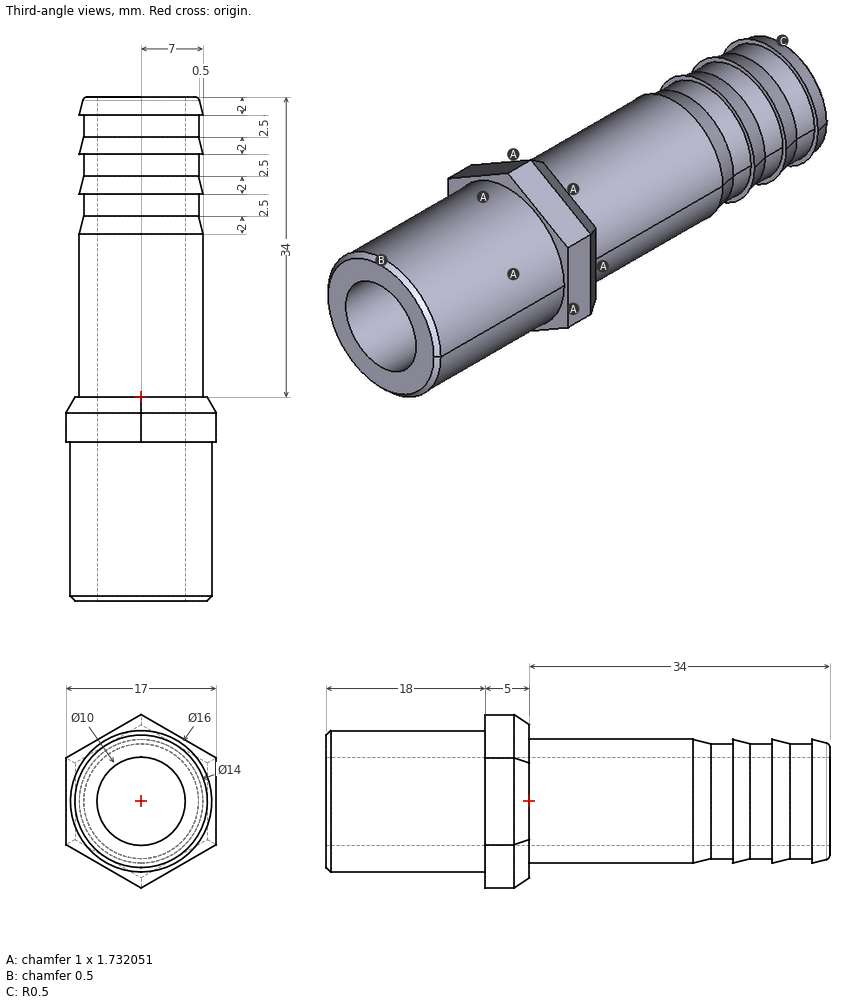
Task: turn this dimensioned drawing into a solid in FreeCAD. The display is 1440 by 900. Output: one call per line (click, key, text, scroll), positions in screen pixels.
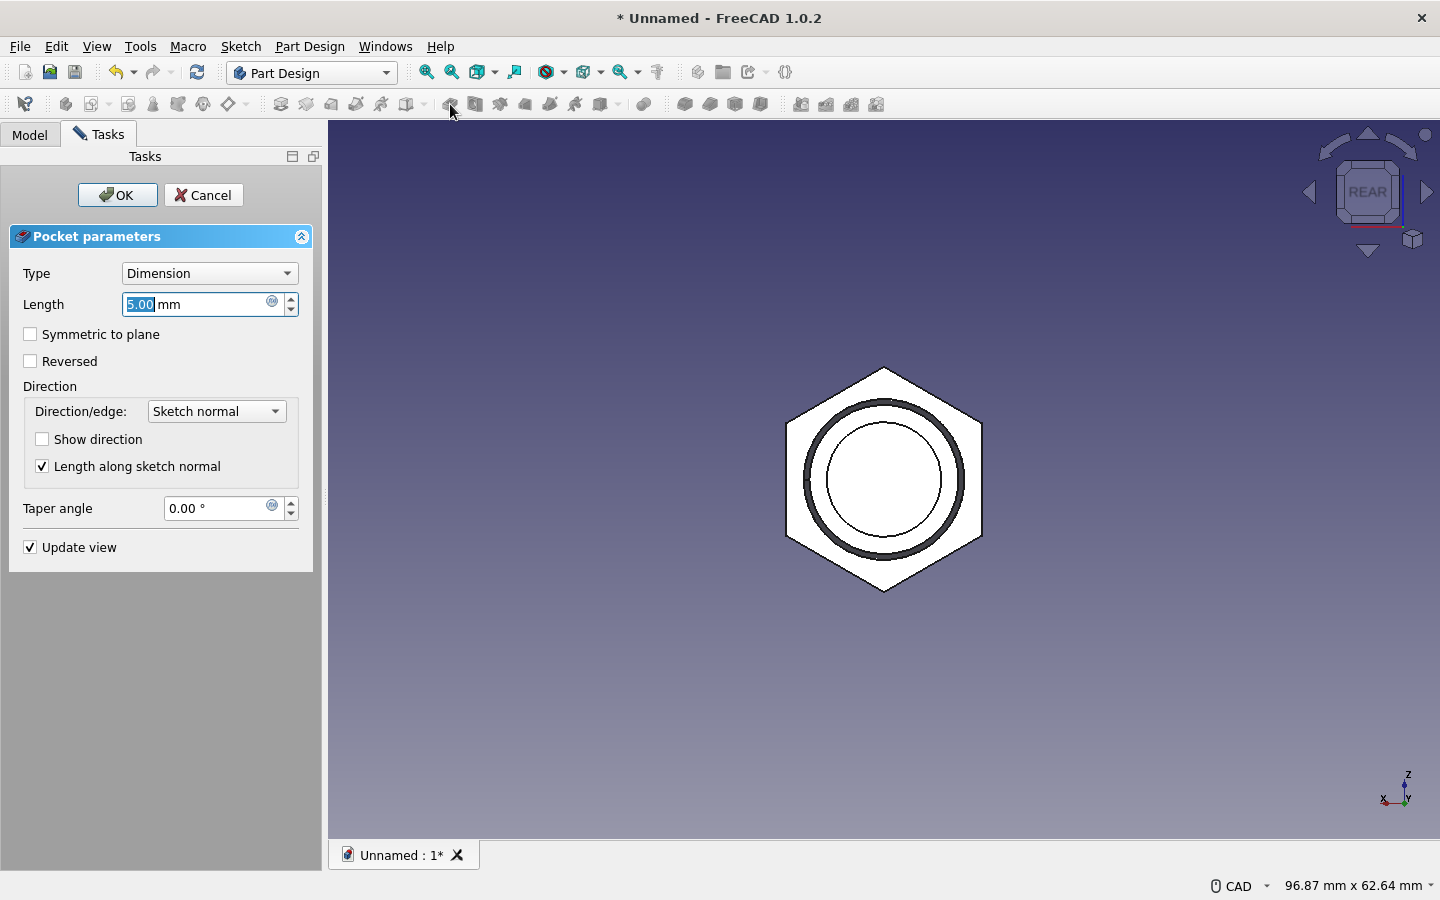
click(210, 274)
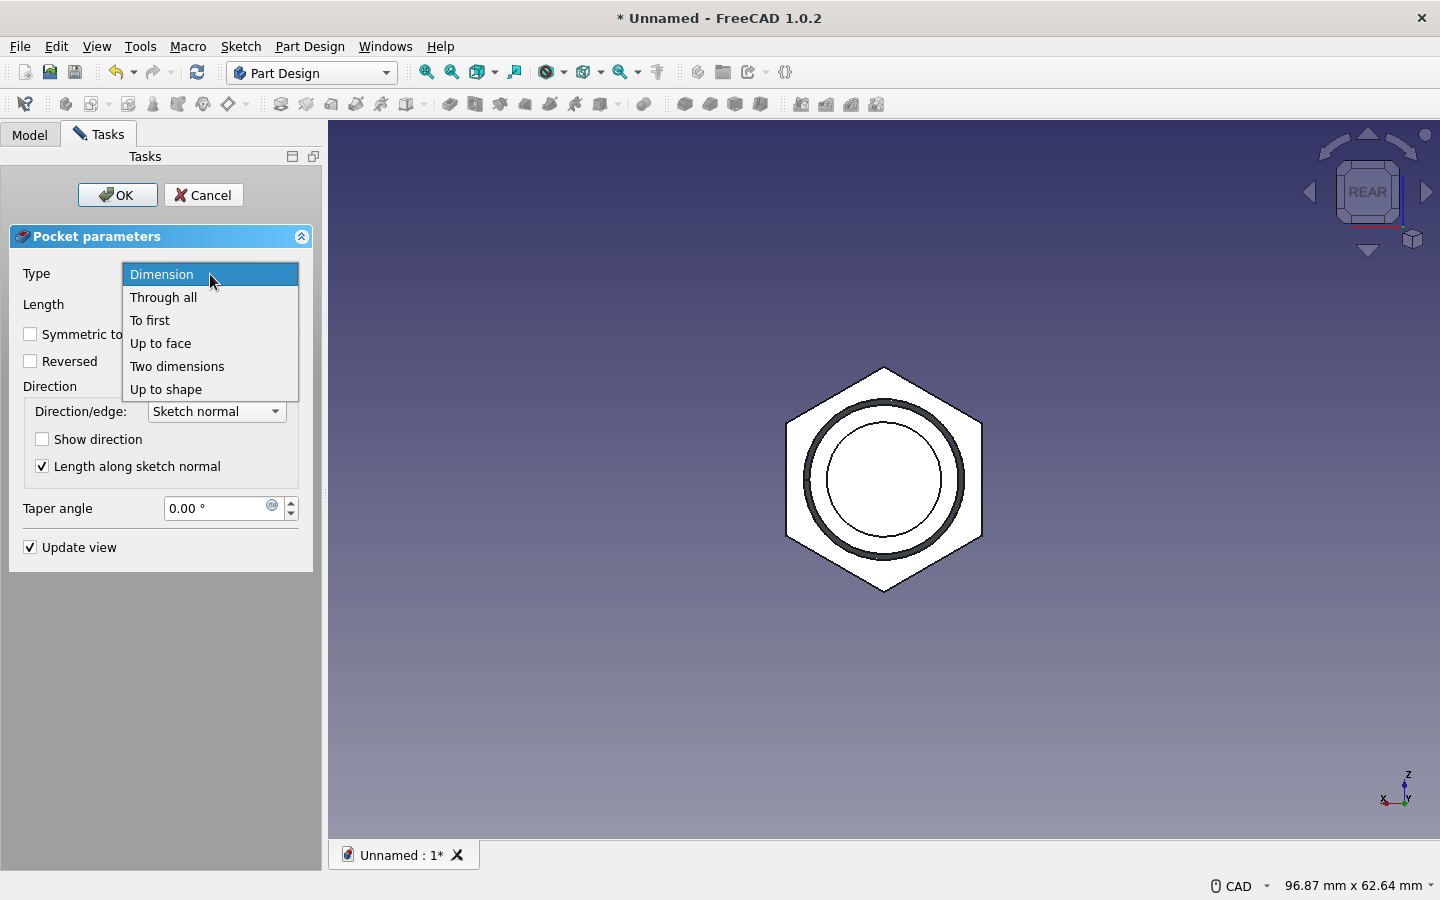
click(208, 298)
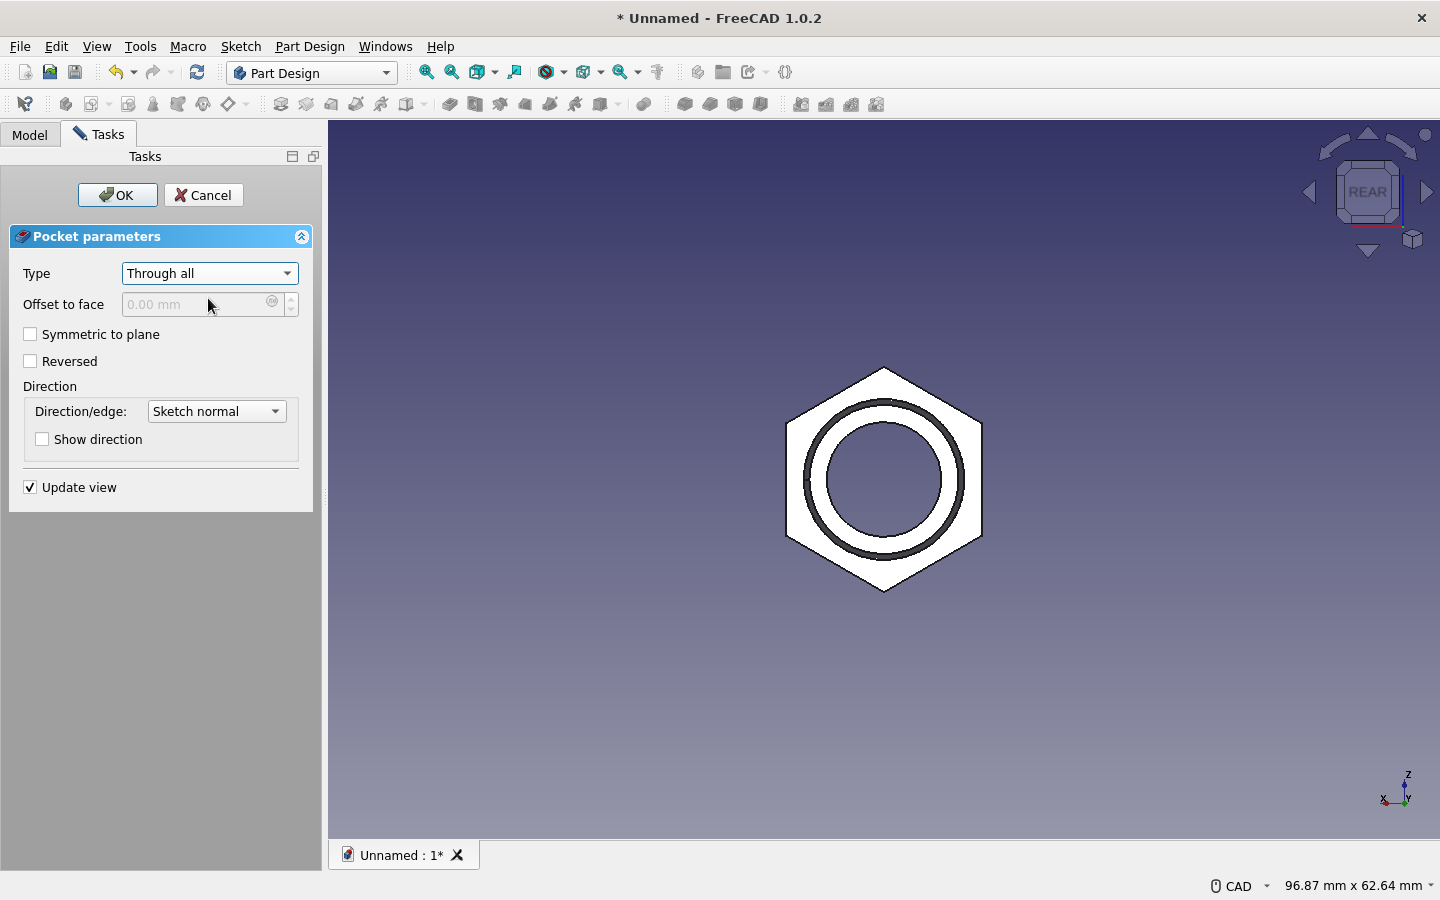
click(118, 195)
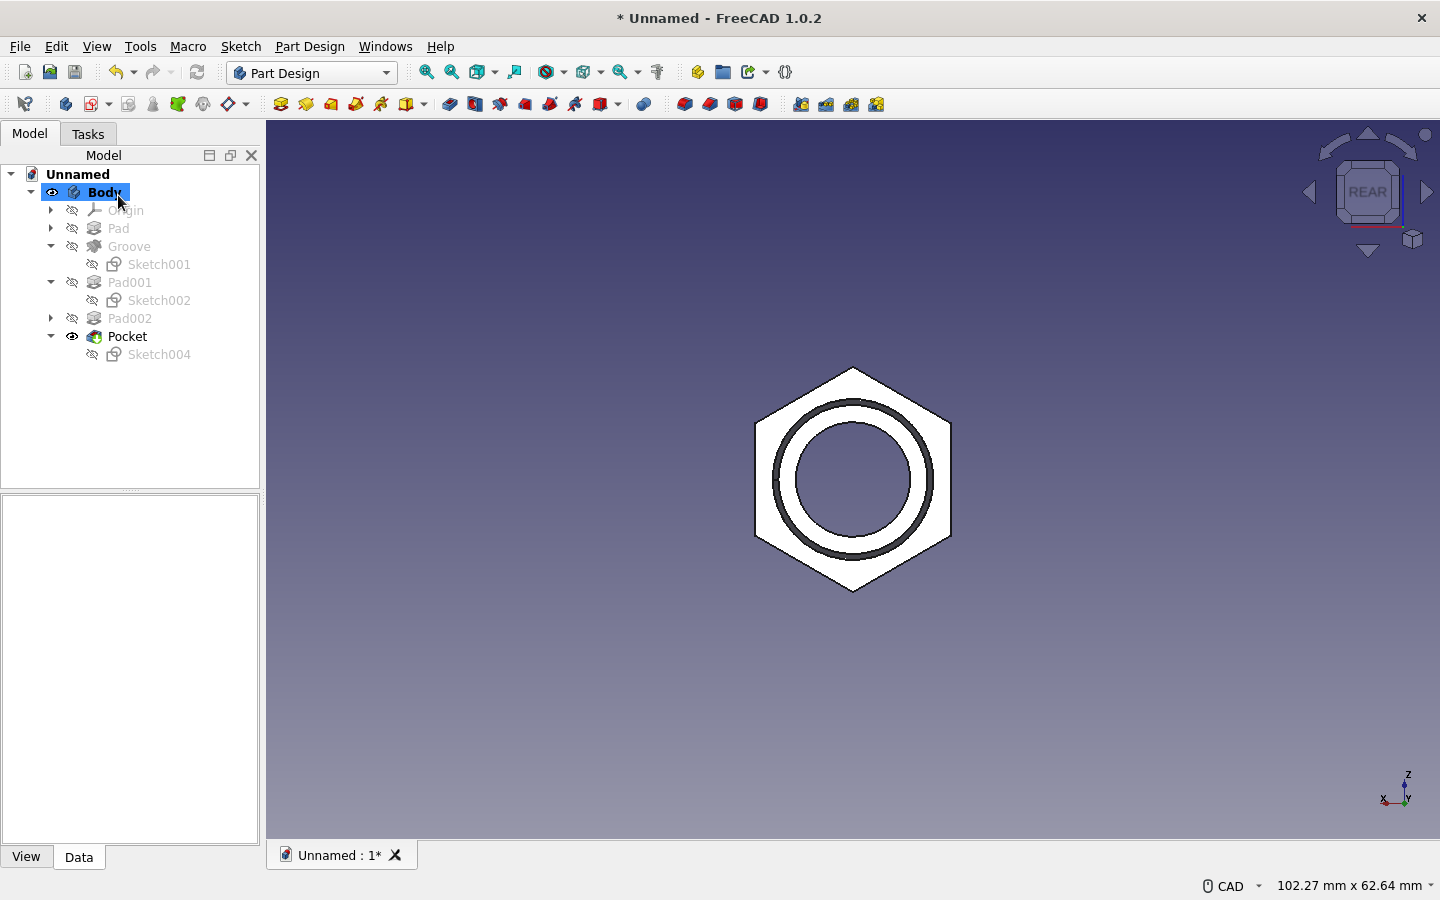
click(427, 72)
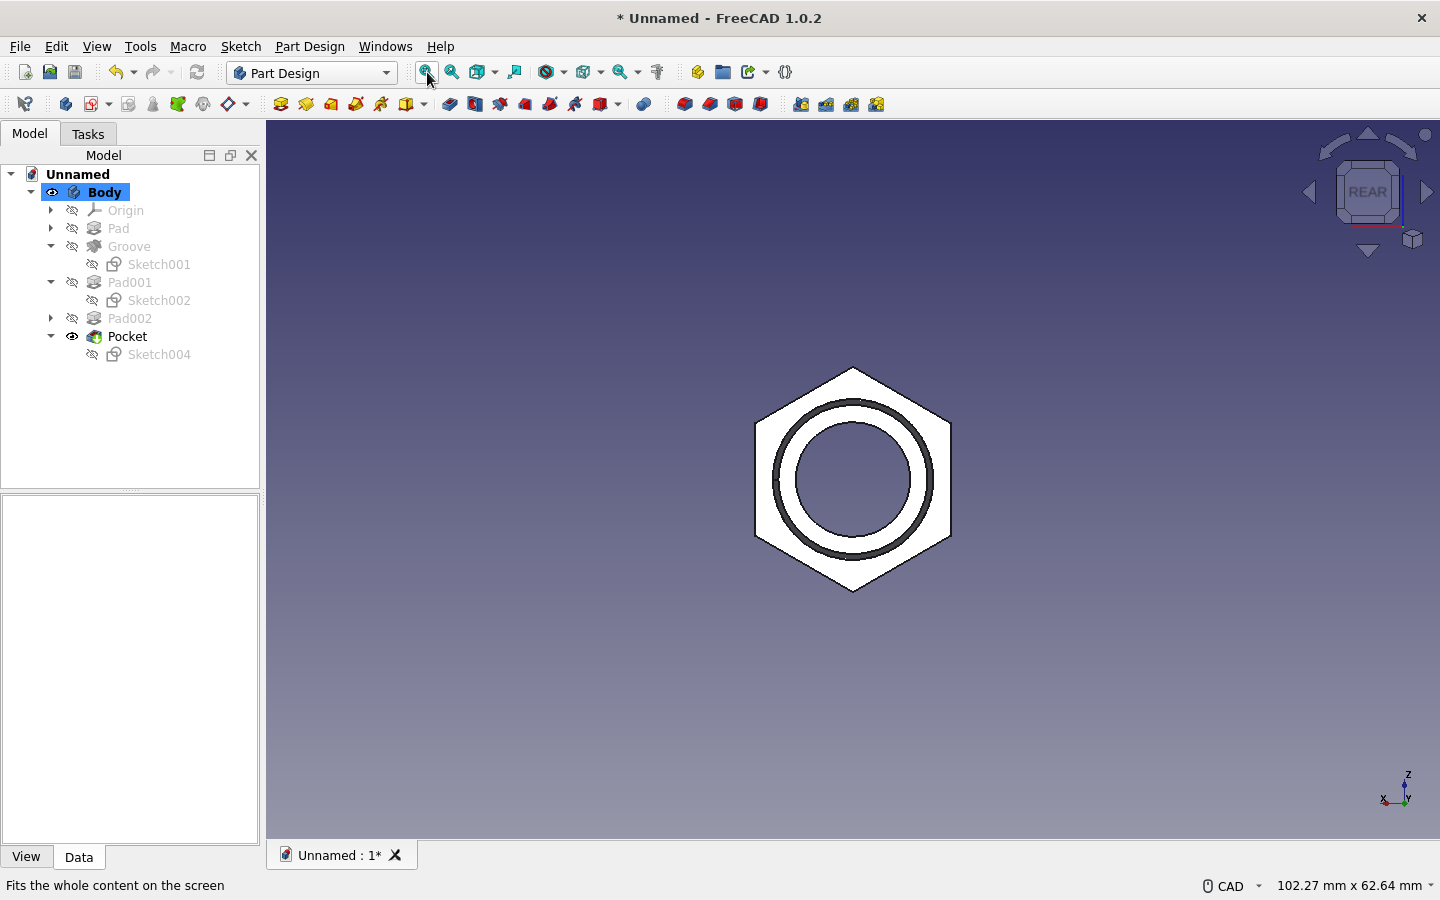
click(804, 563)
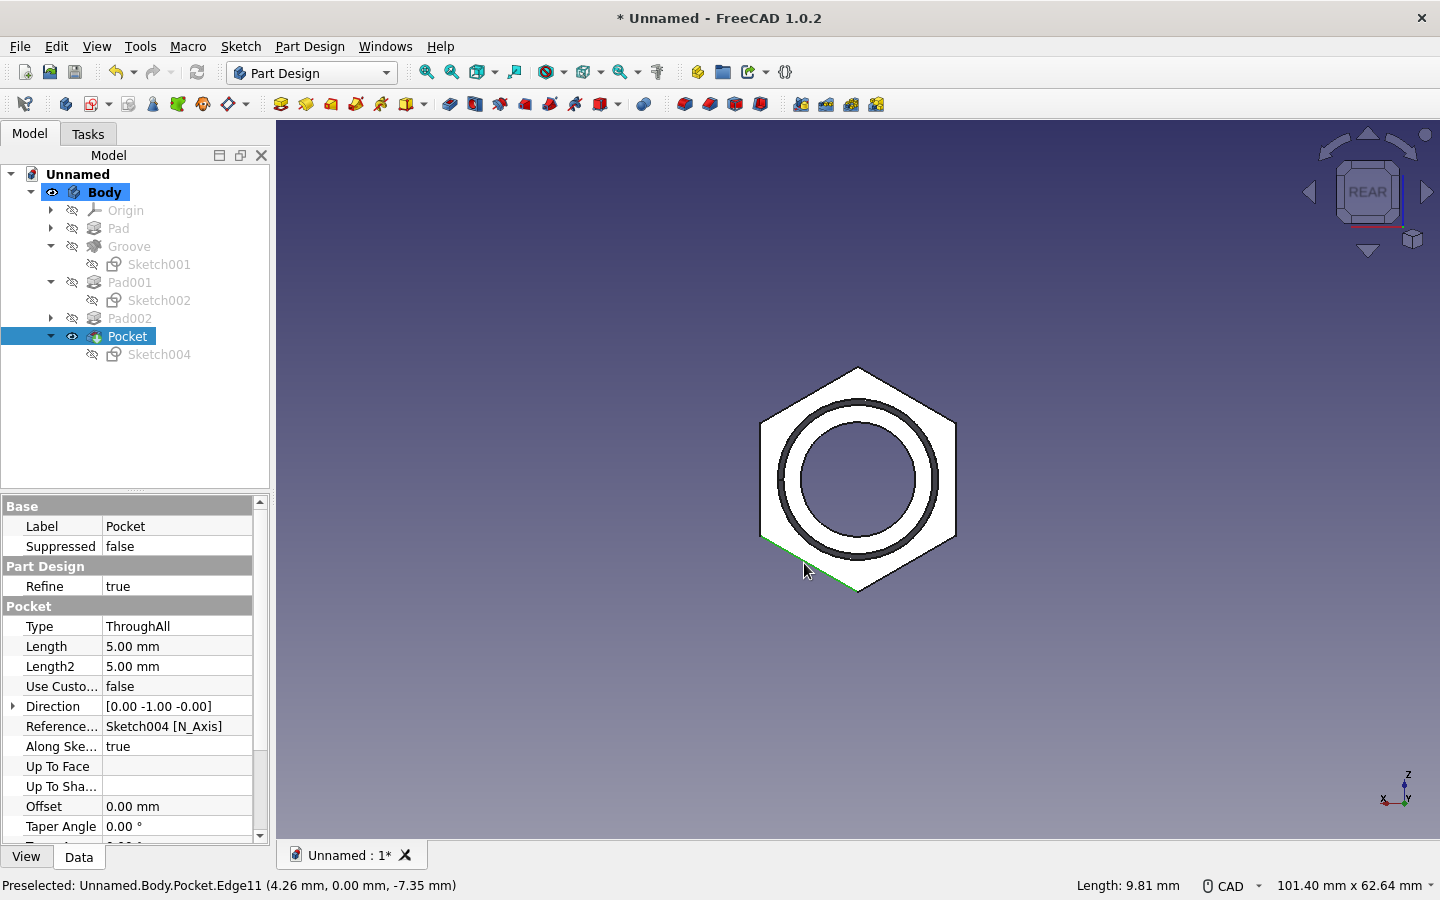
click(956, 478, ctrl)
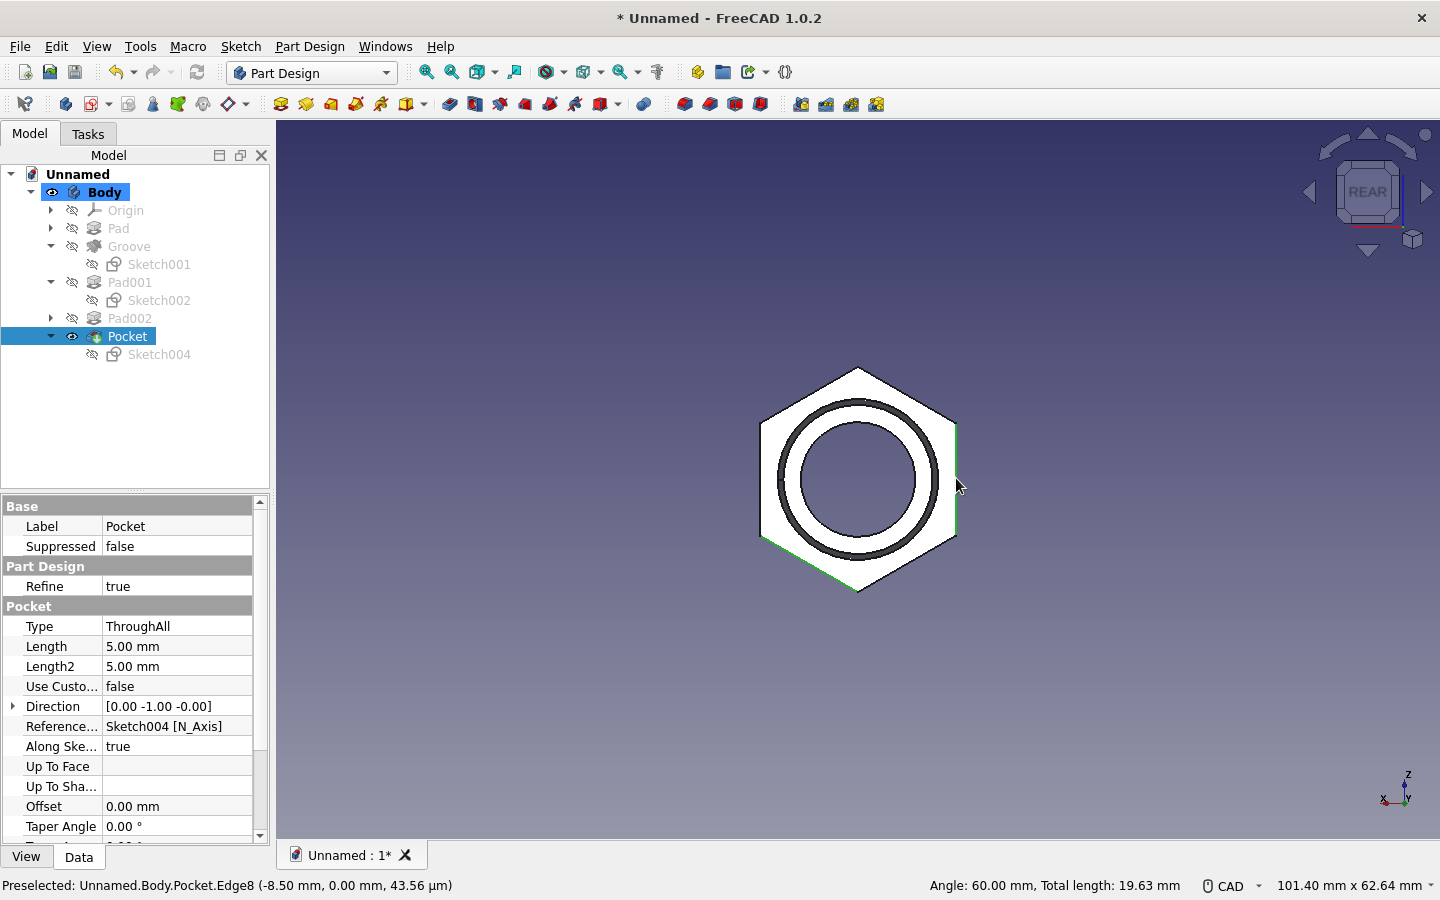
click(907, 563, ctrl)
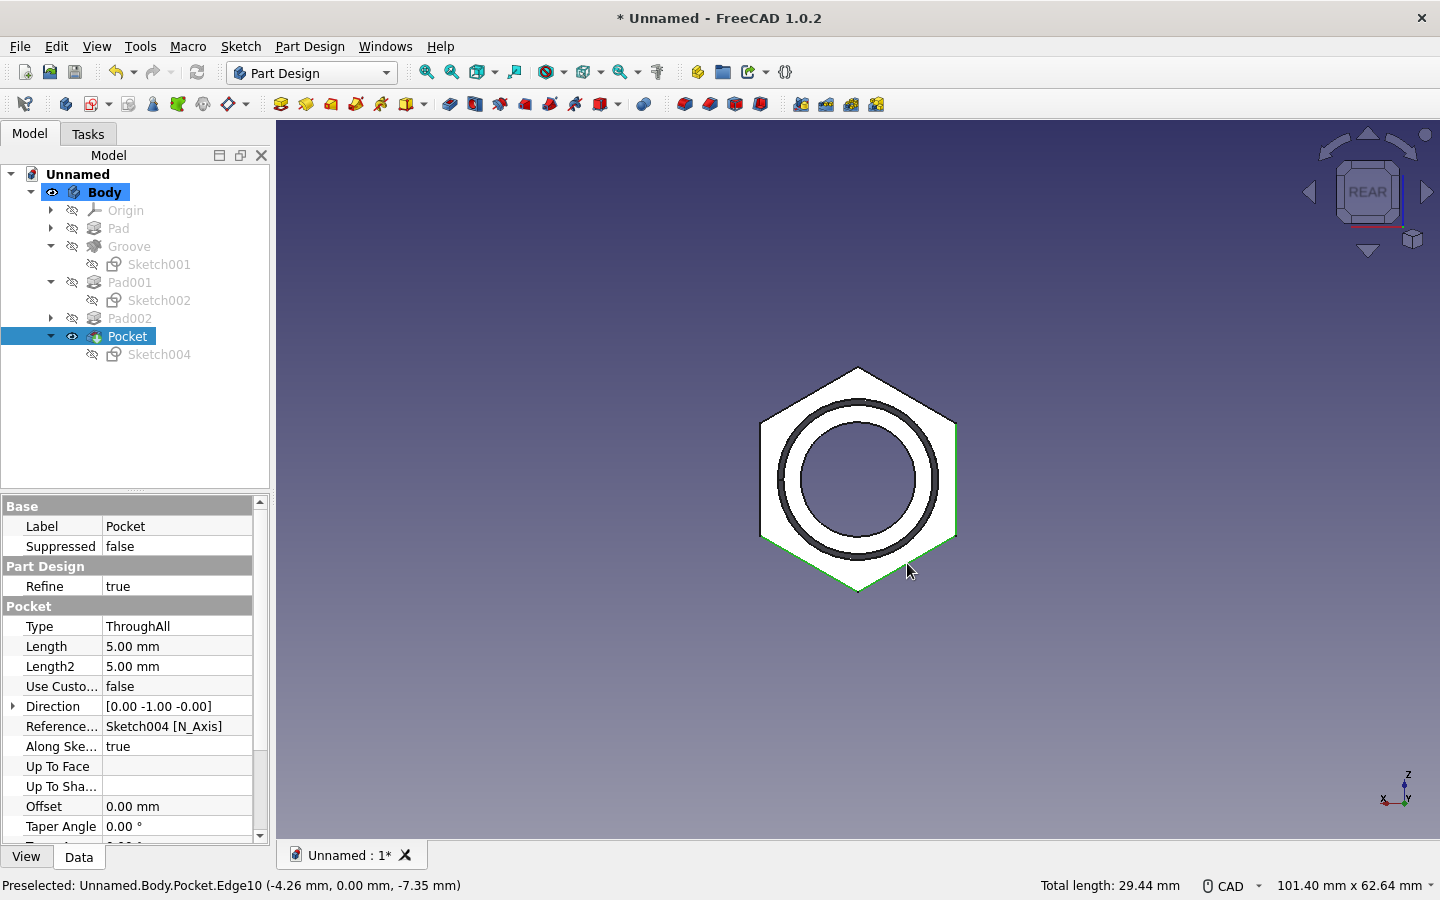
key(0)